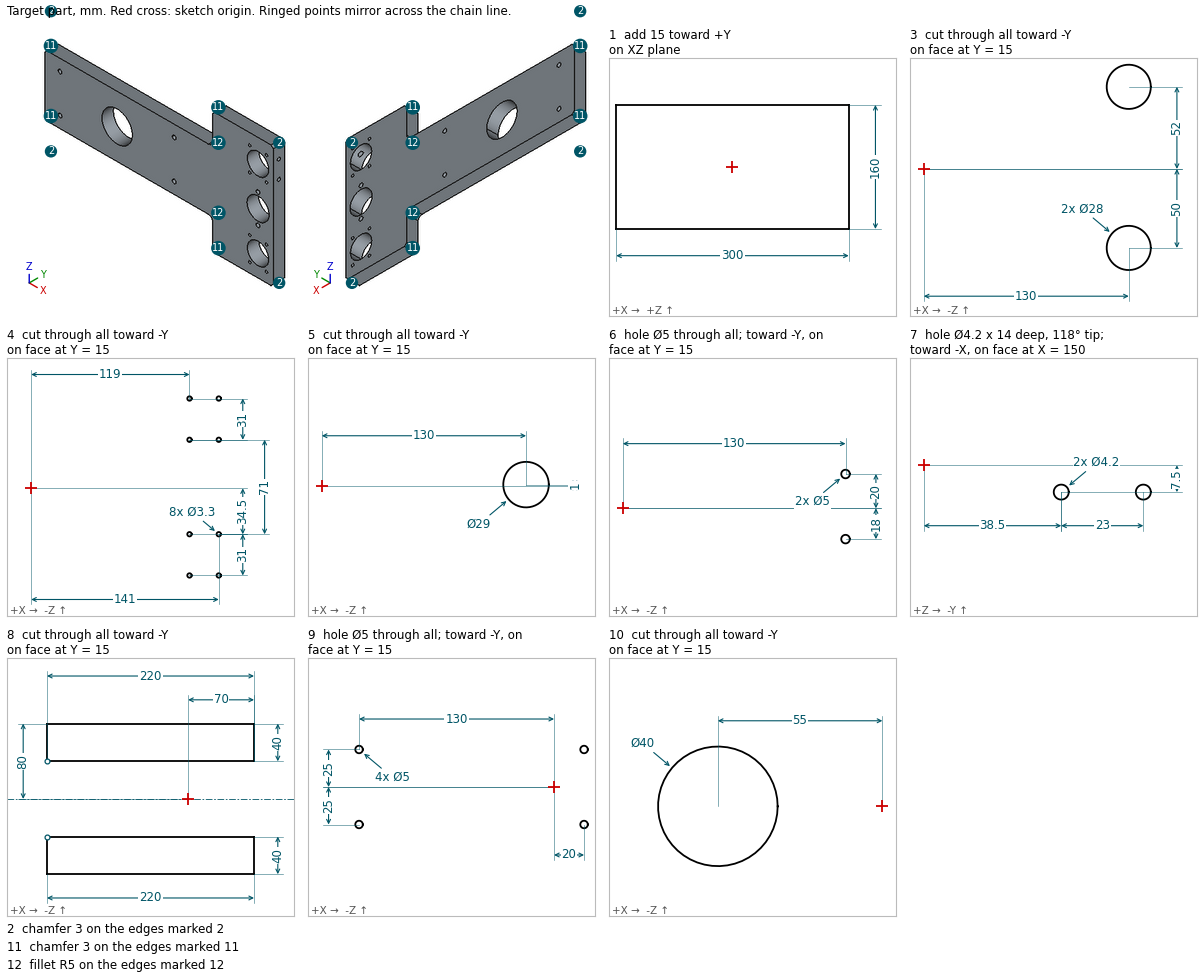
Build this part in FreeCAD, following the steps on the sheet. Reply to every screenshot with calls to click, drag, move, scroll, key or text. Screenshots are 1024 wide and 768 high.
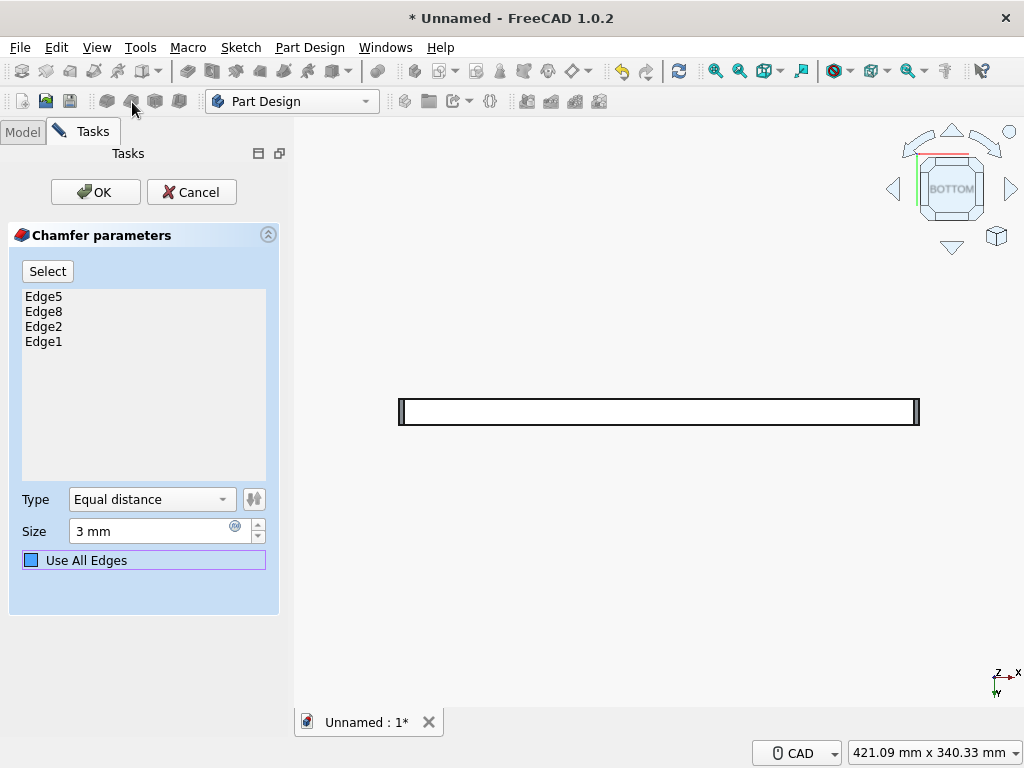
click(96, 192)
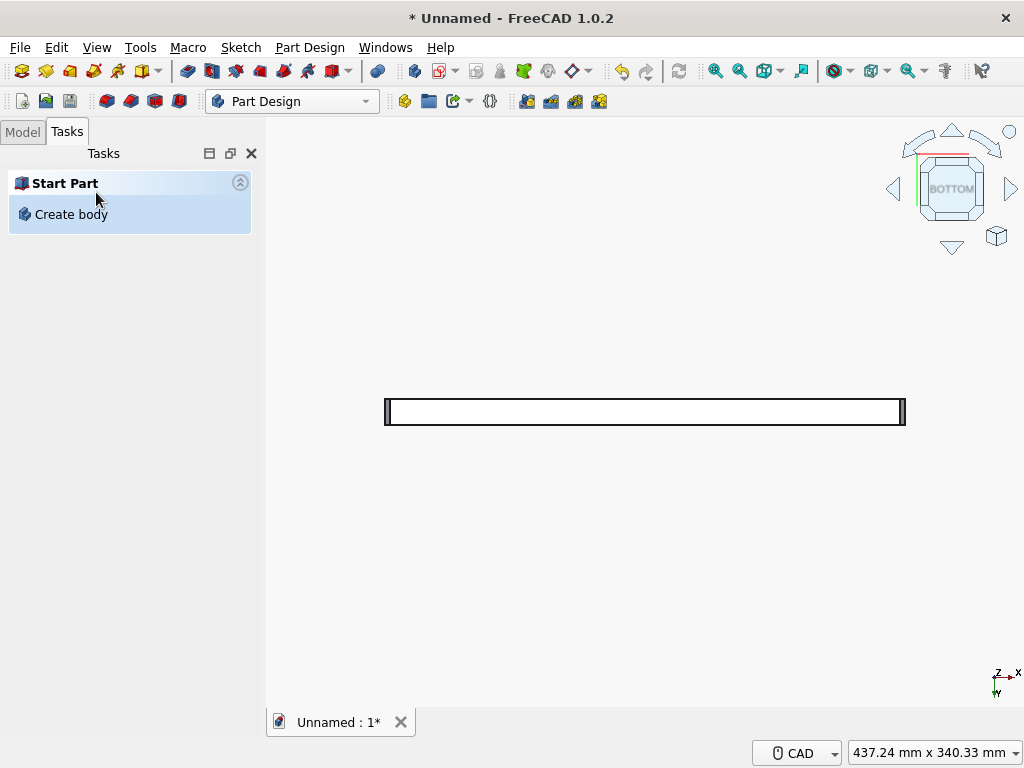
key(4)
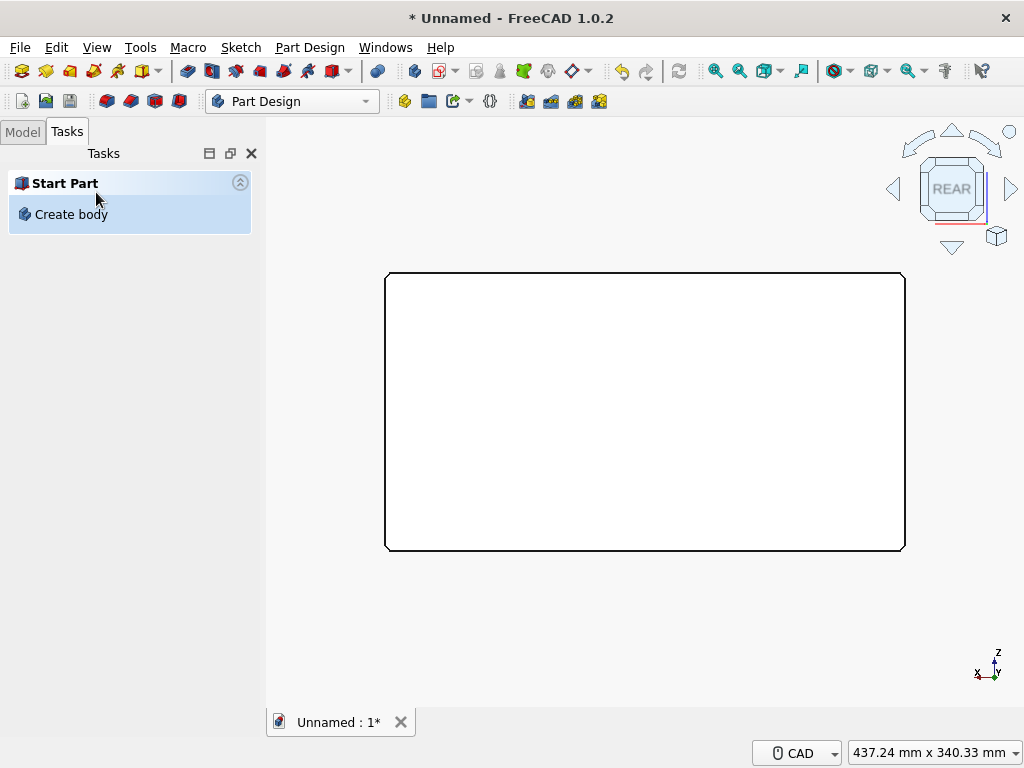
click(571, 411)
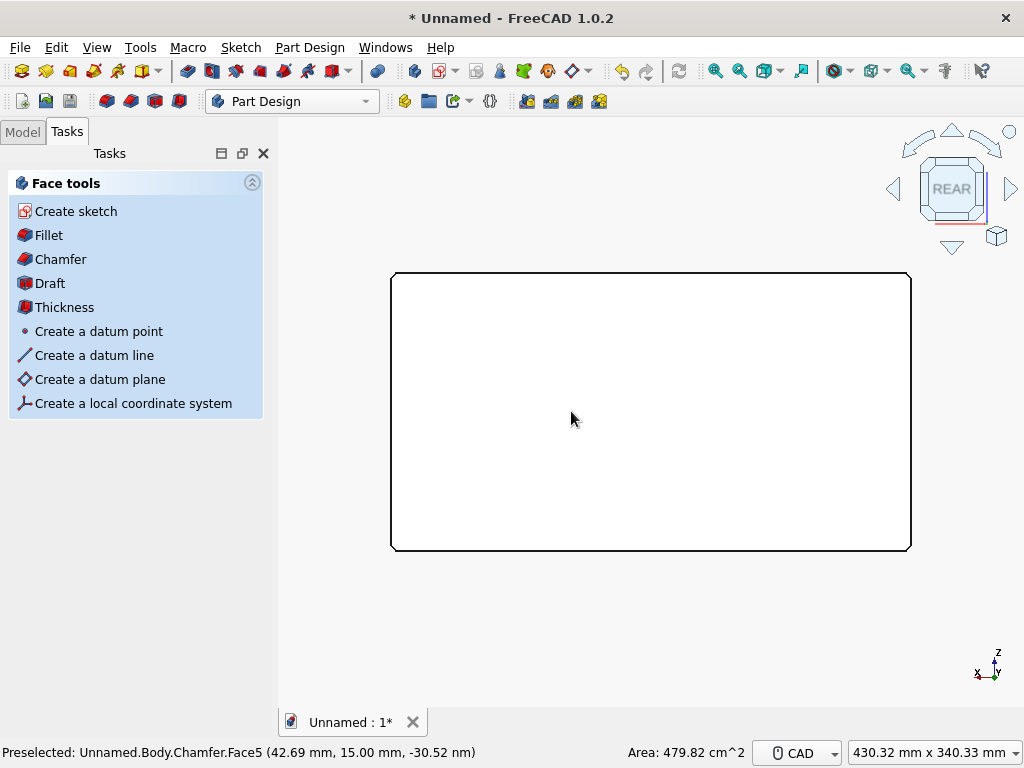
click(440, 72)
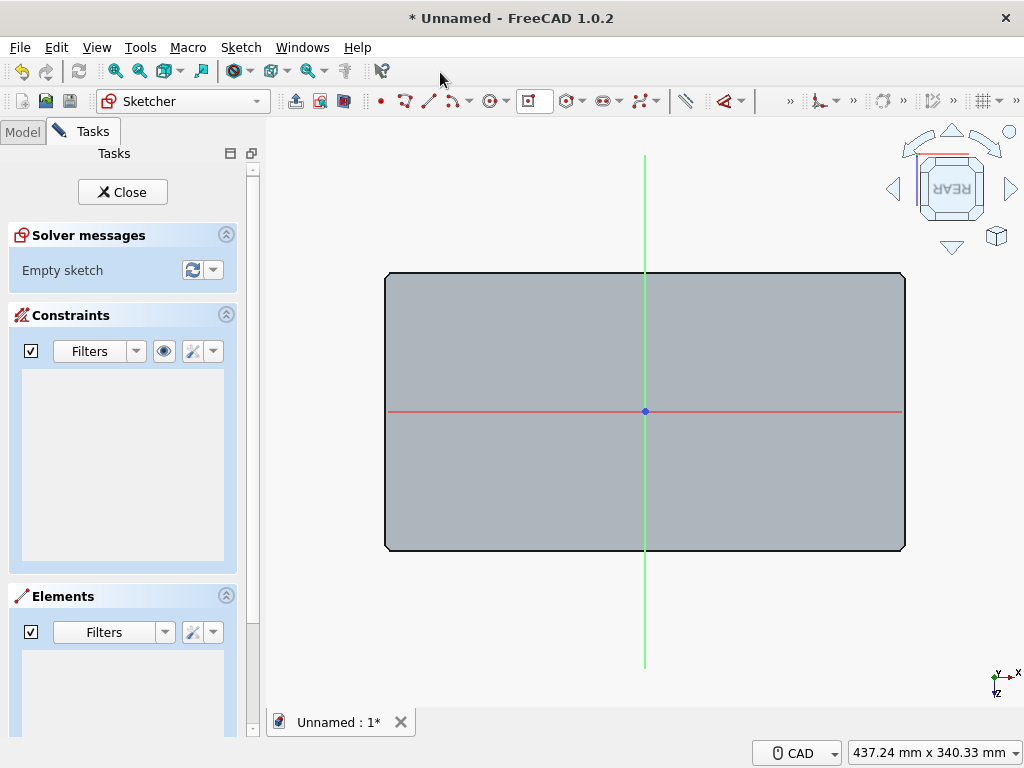
scroll(294, 420, down, 1)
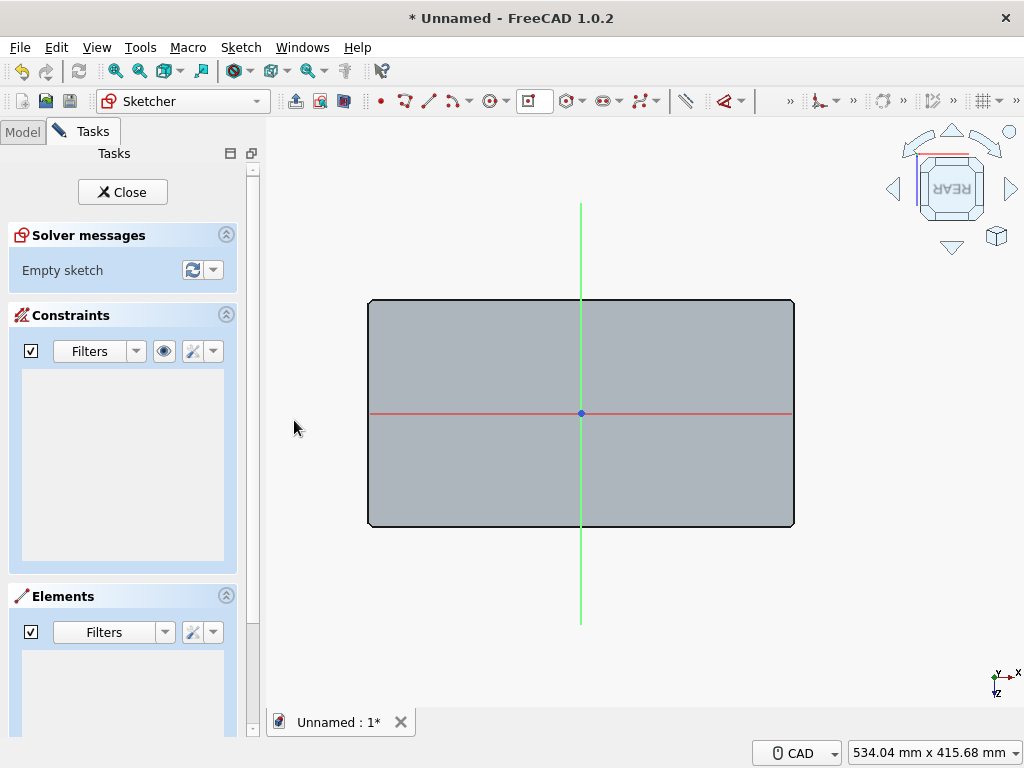
scroll(814, 412, up, 3)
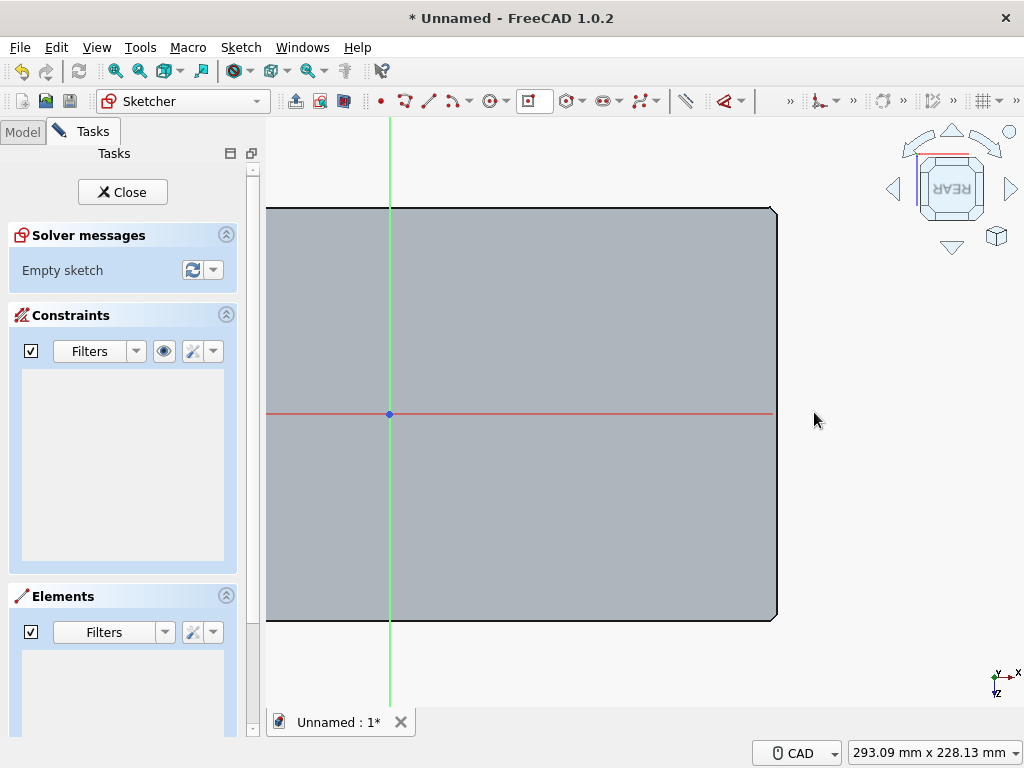
click(490, 102)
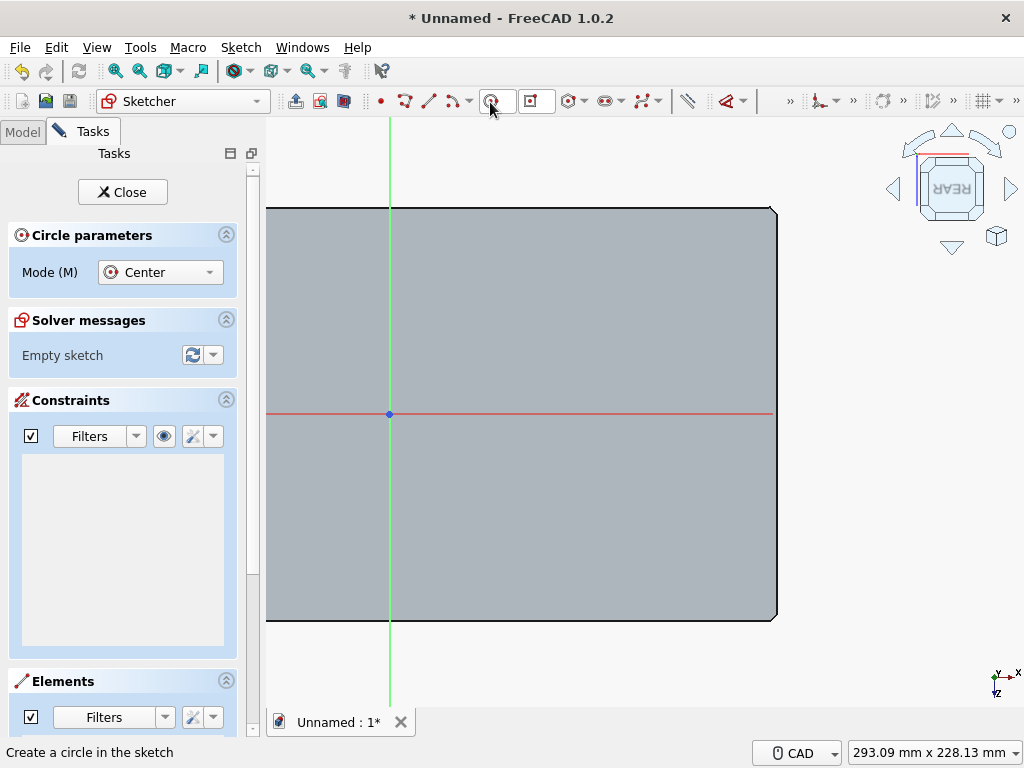
click(726, 544)
move(751, 518)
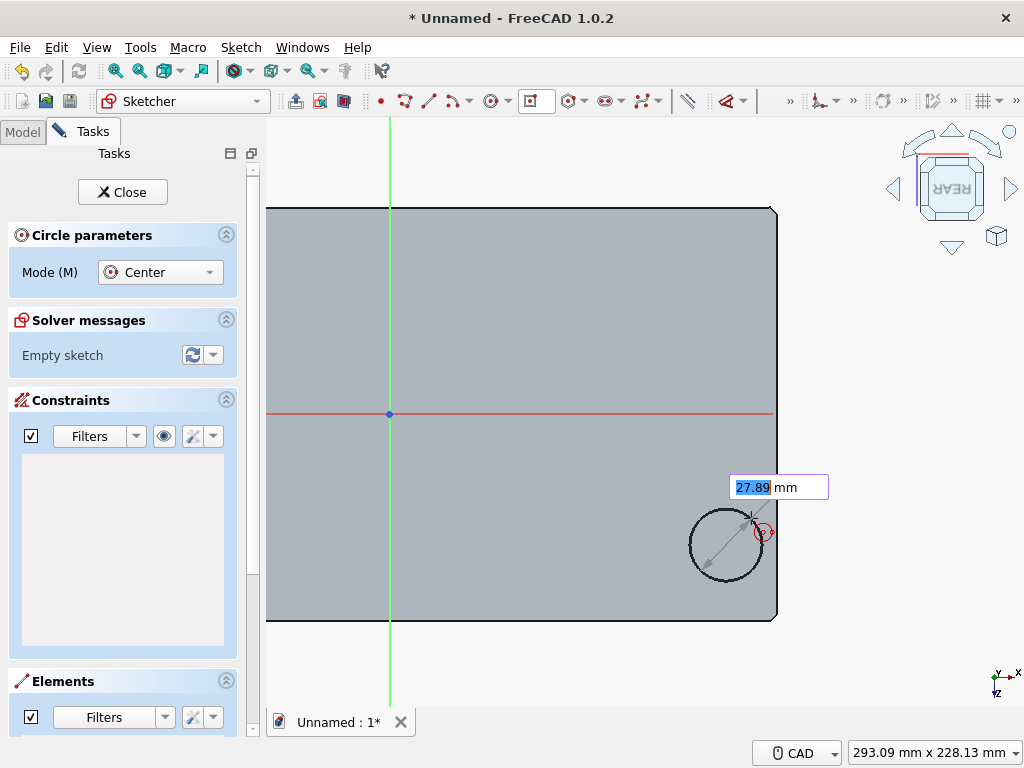
text(28)
key(Return)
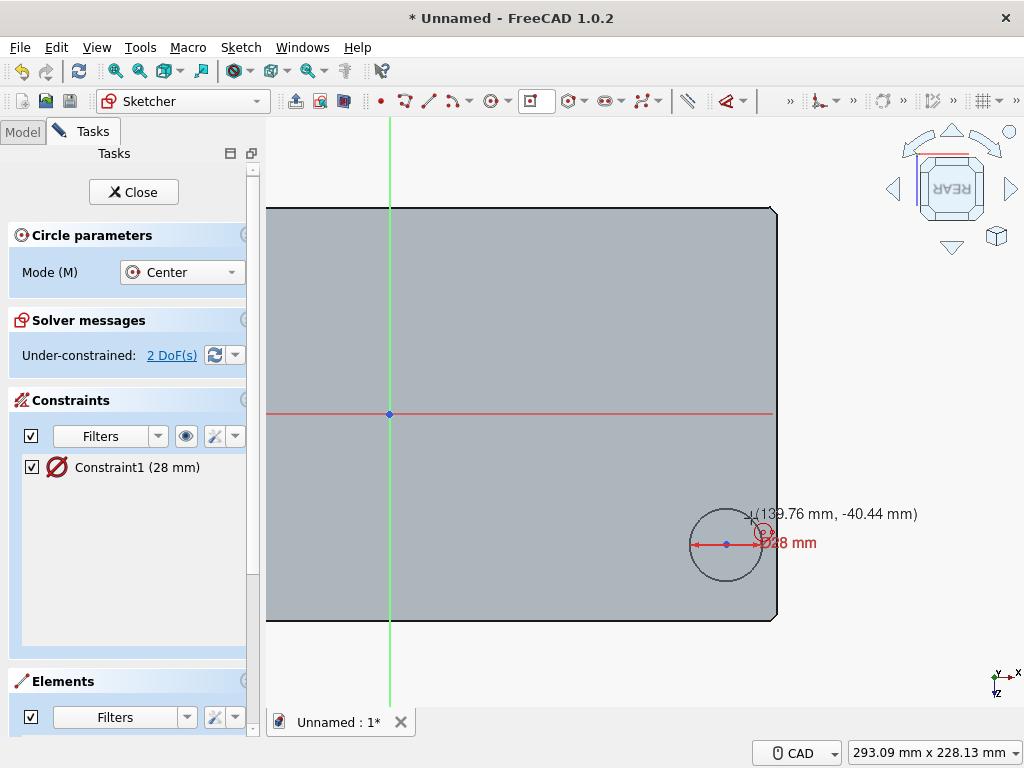
click(726, 280)
move(751, 254)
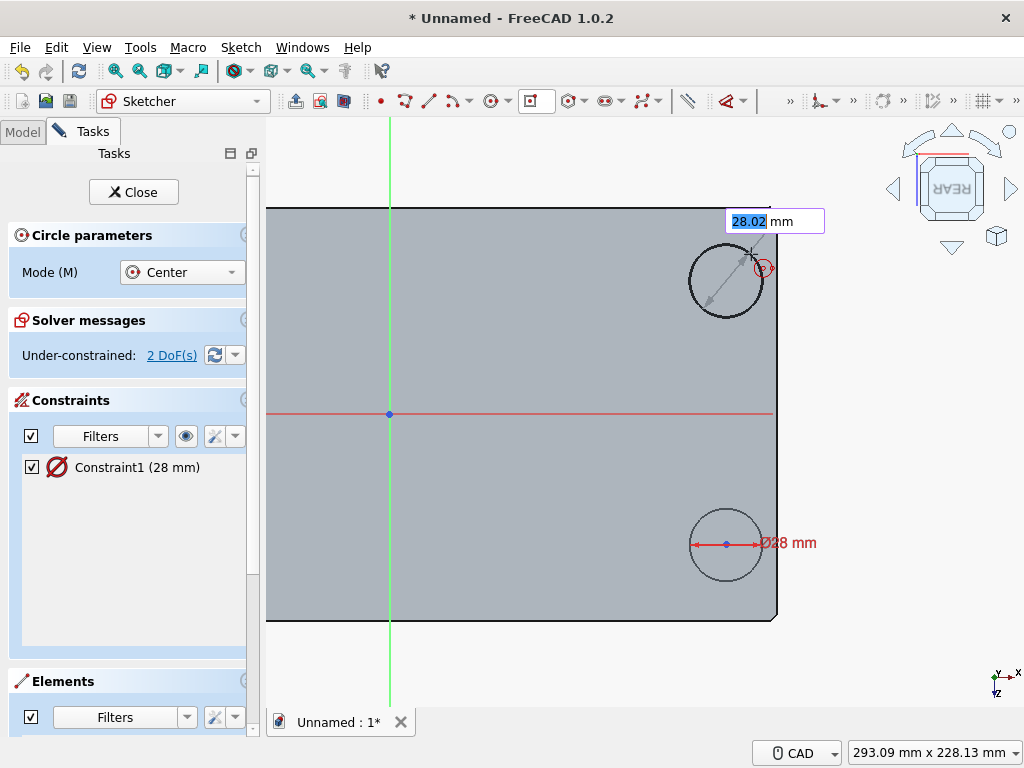
text(28)
key(Return)
key(Escape)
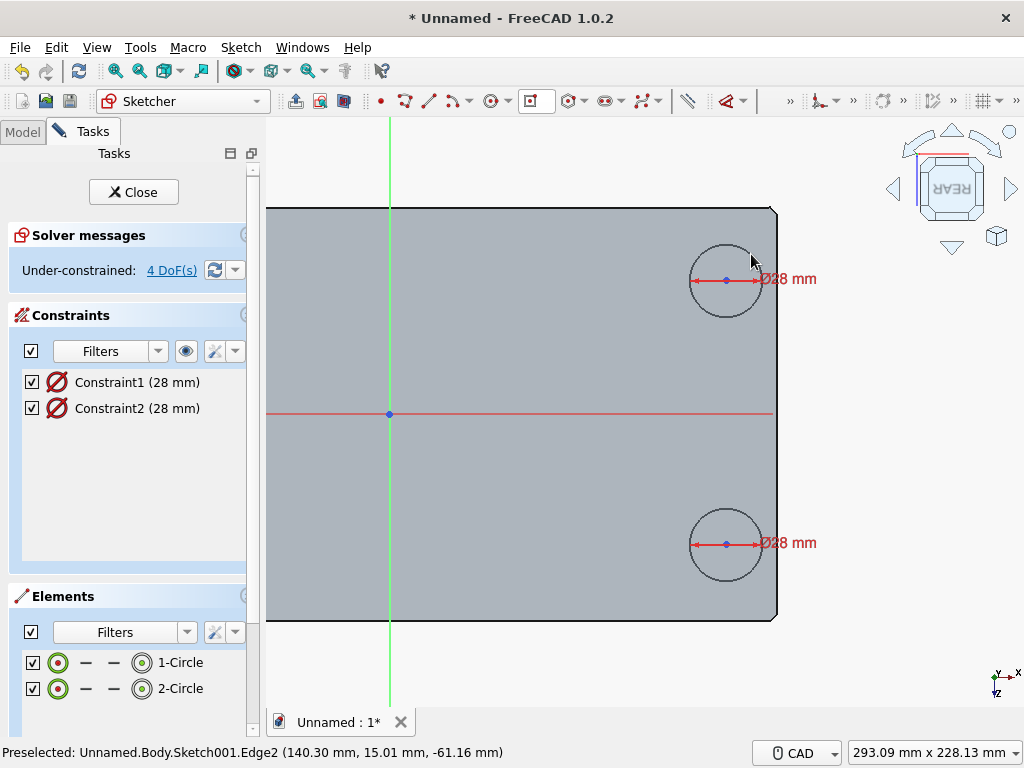
click(726, 545)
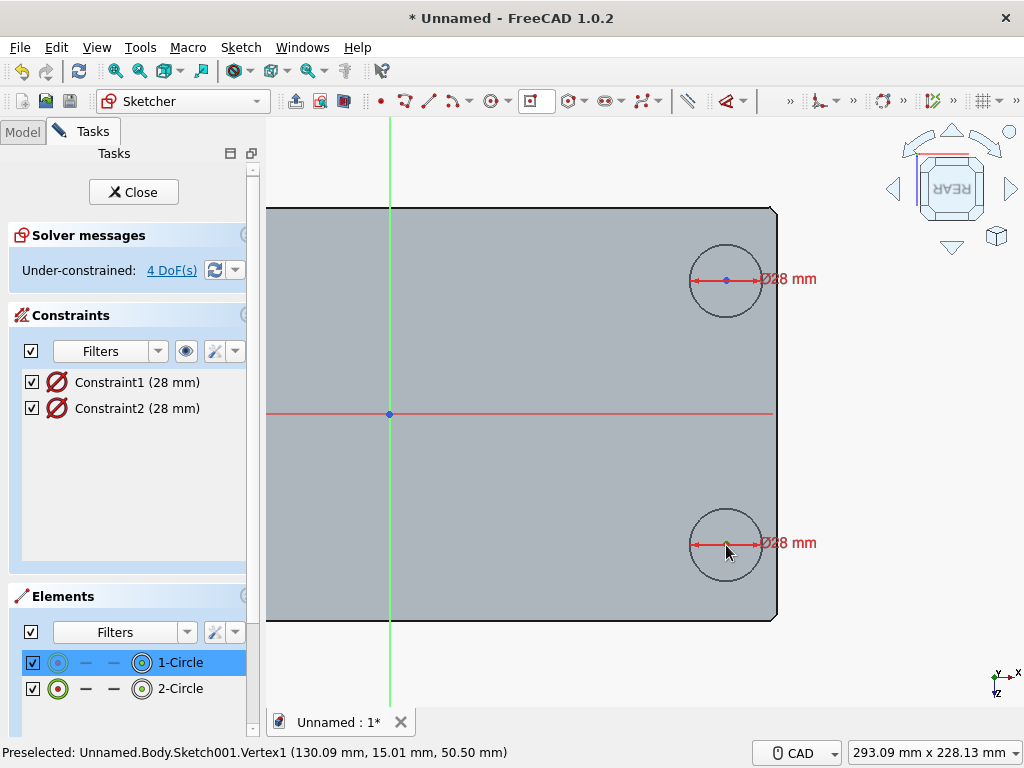
click(726, 281)